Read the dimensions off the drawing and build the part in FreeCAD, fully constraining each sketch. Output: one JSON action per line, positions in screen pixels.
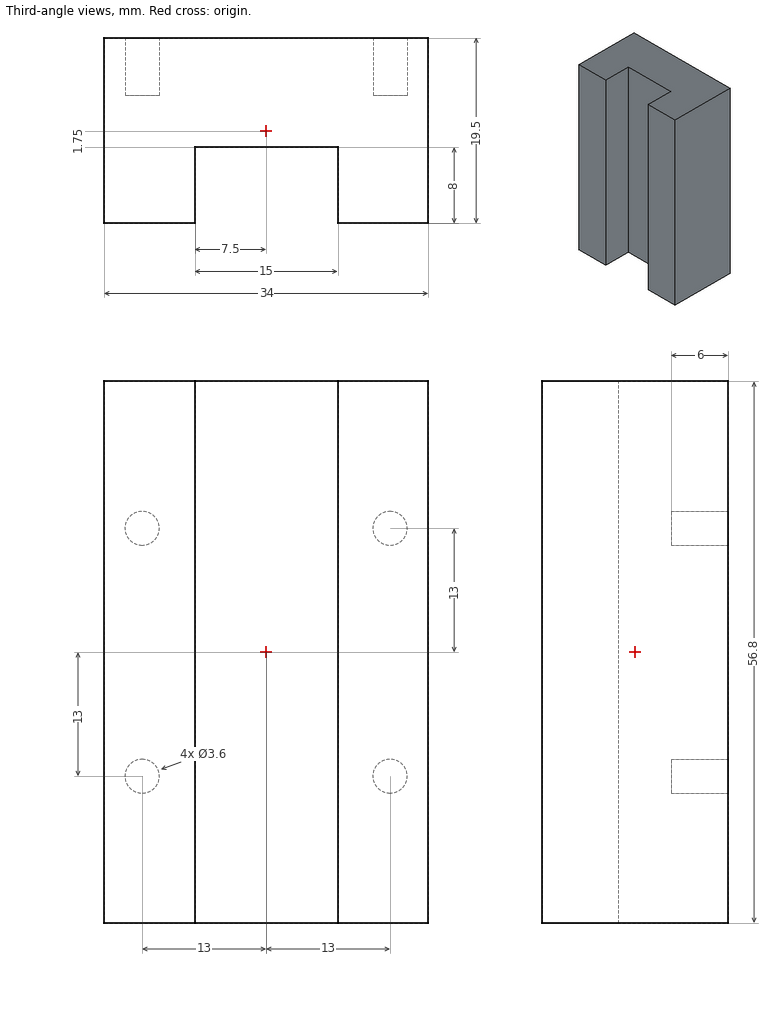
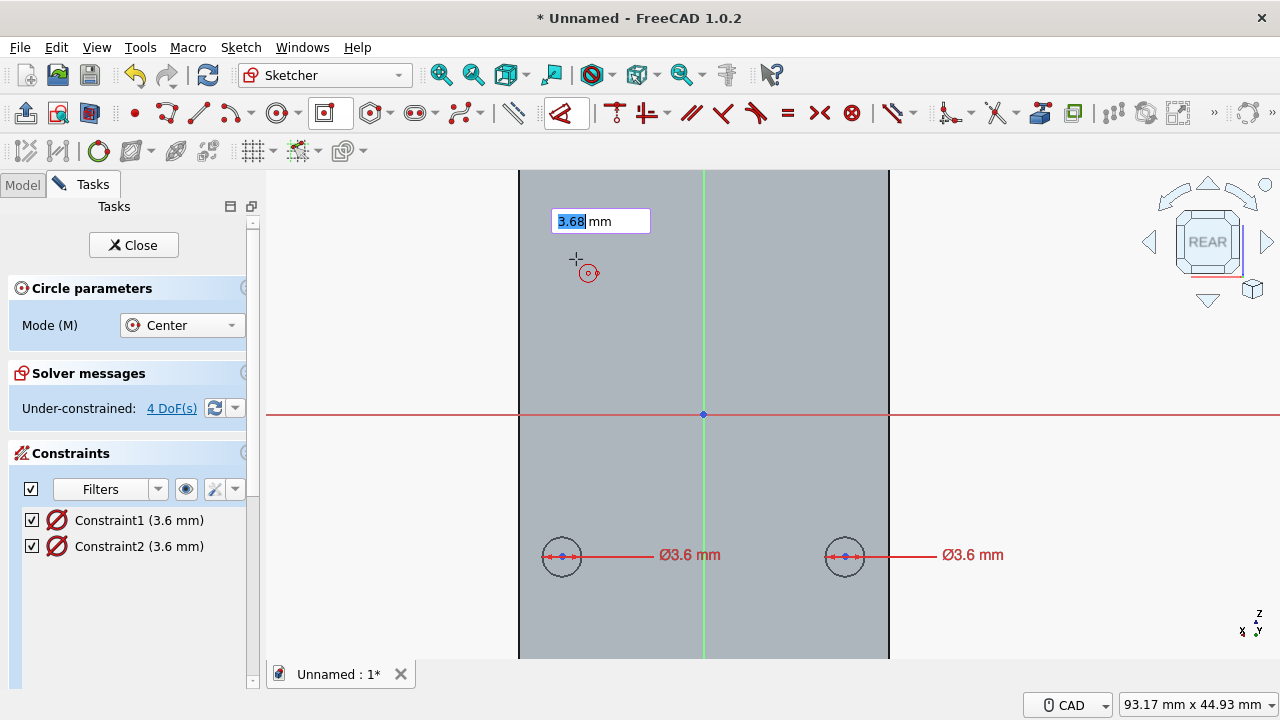
{"action": "type", "text": "3.6"}
{"action": "key", "text": "Return"}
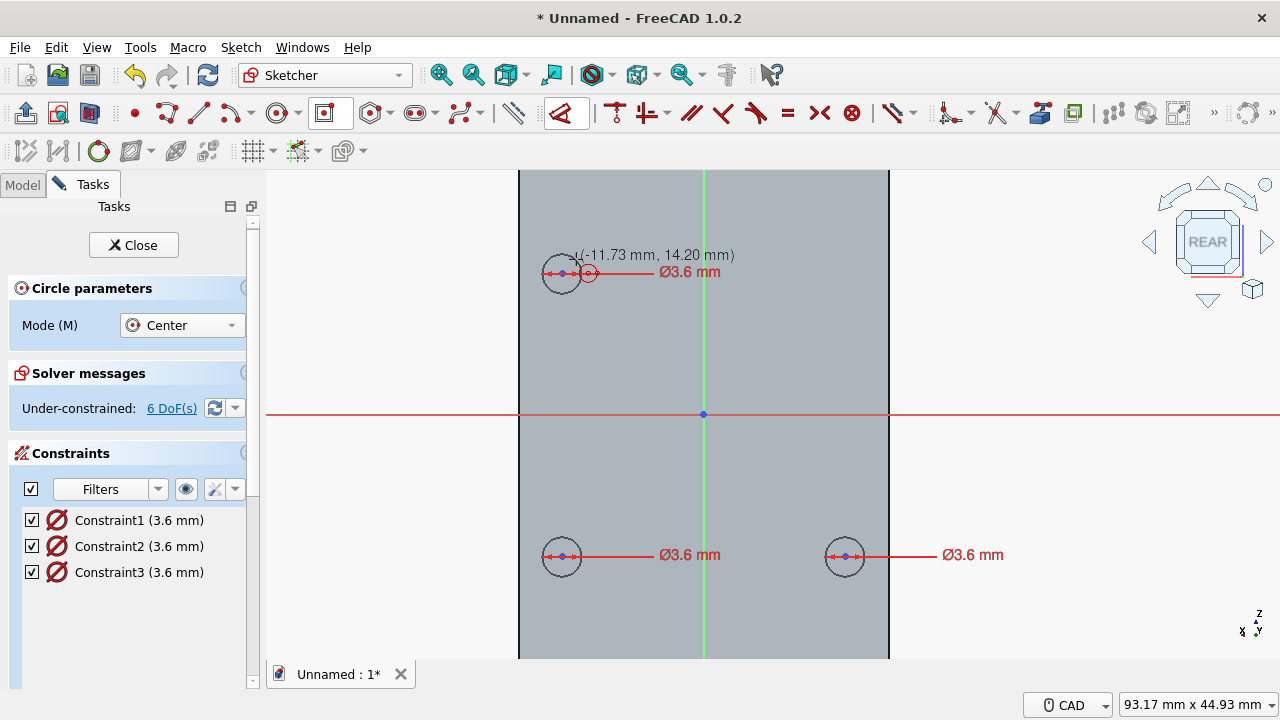
{"action": "left_click", "coordinate": [845, 273]}
{"action": "mouse_move", "coordinate": [859, 259]}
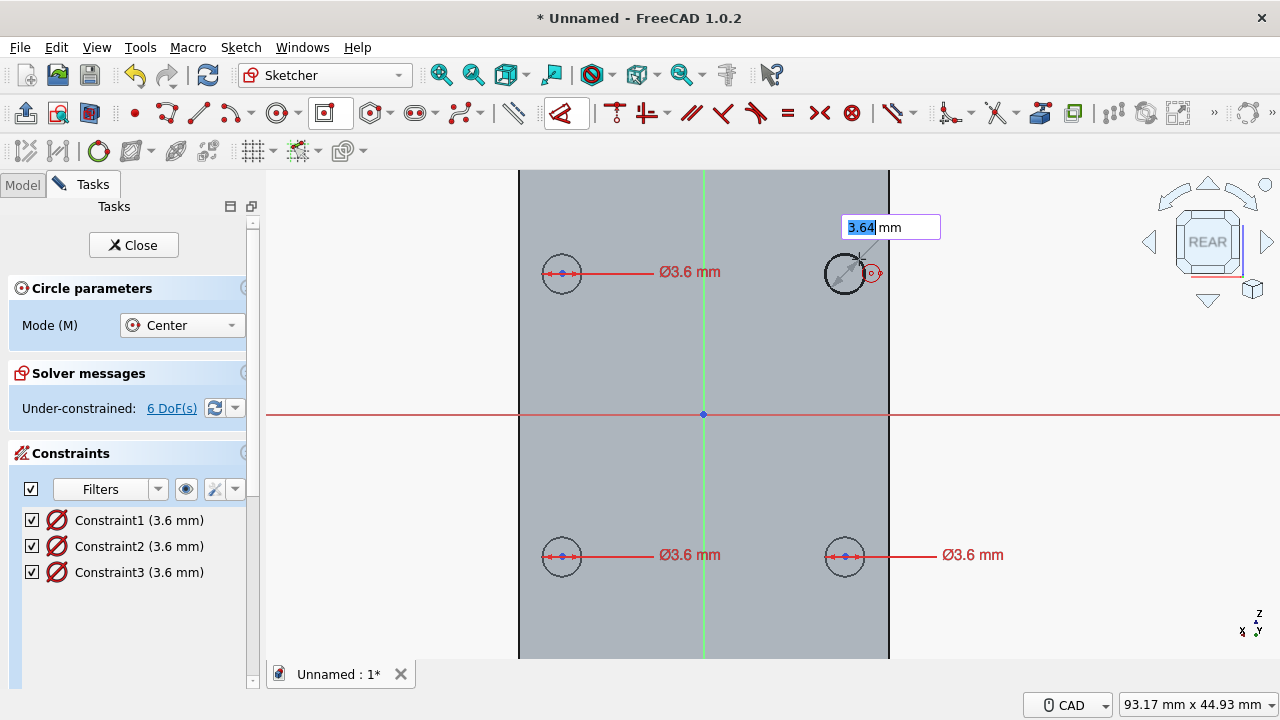
{"action": "type", "text": "3.6"}
{"action": "key", "text": "Return"}
{"action": "key", "text": "Escape"}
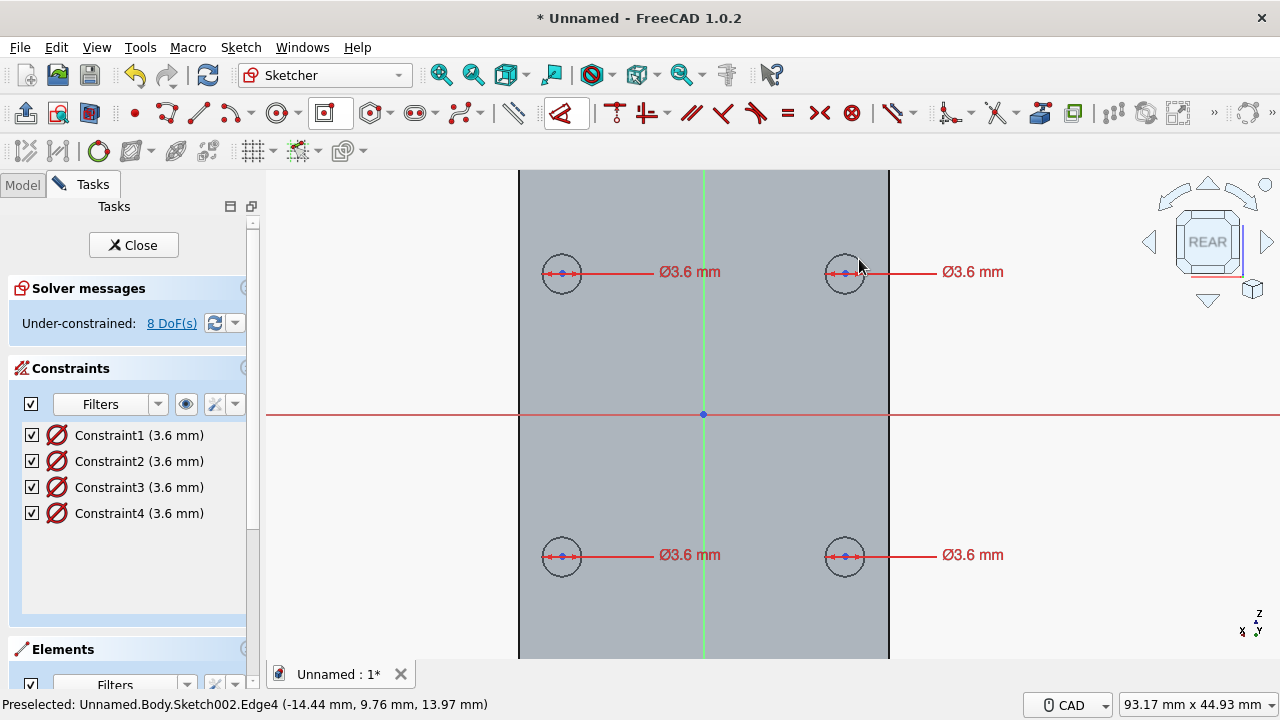
{"action": "left_click", "coordinate": [845, 557]}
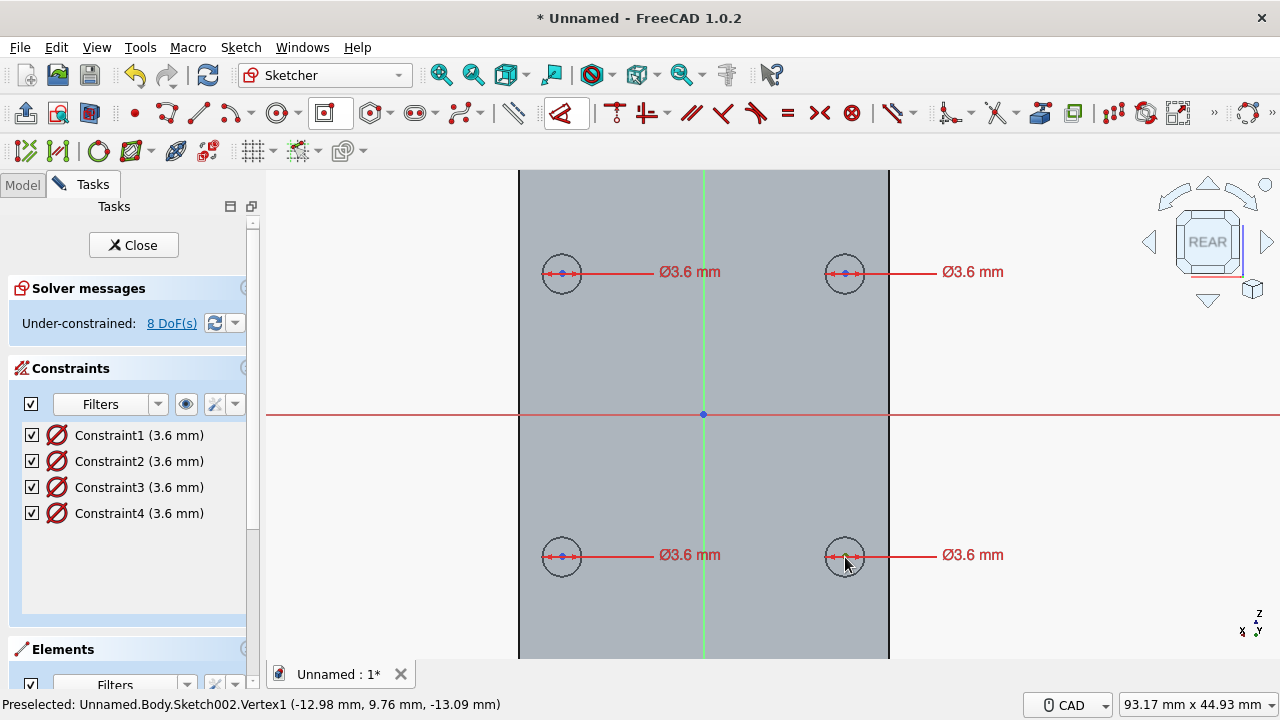
{"action": "left_click", "coordinate": [562, 557]}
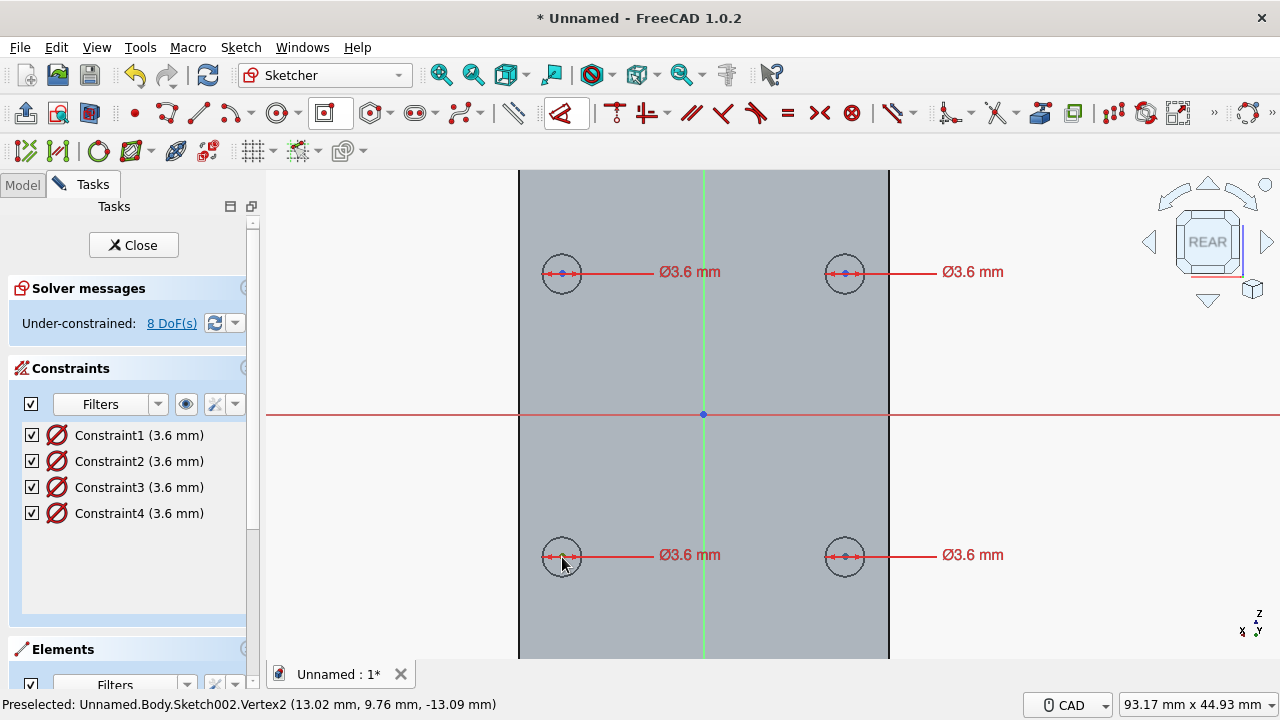
{"action": "left_click", "coordinate": [670, 114]}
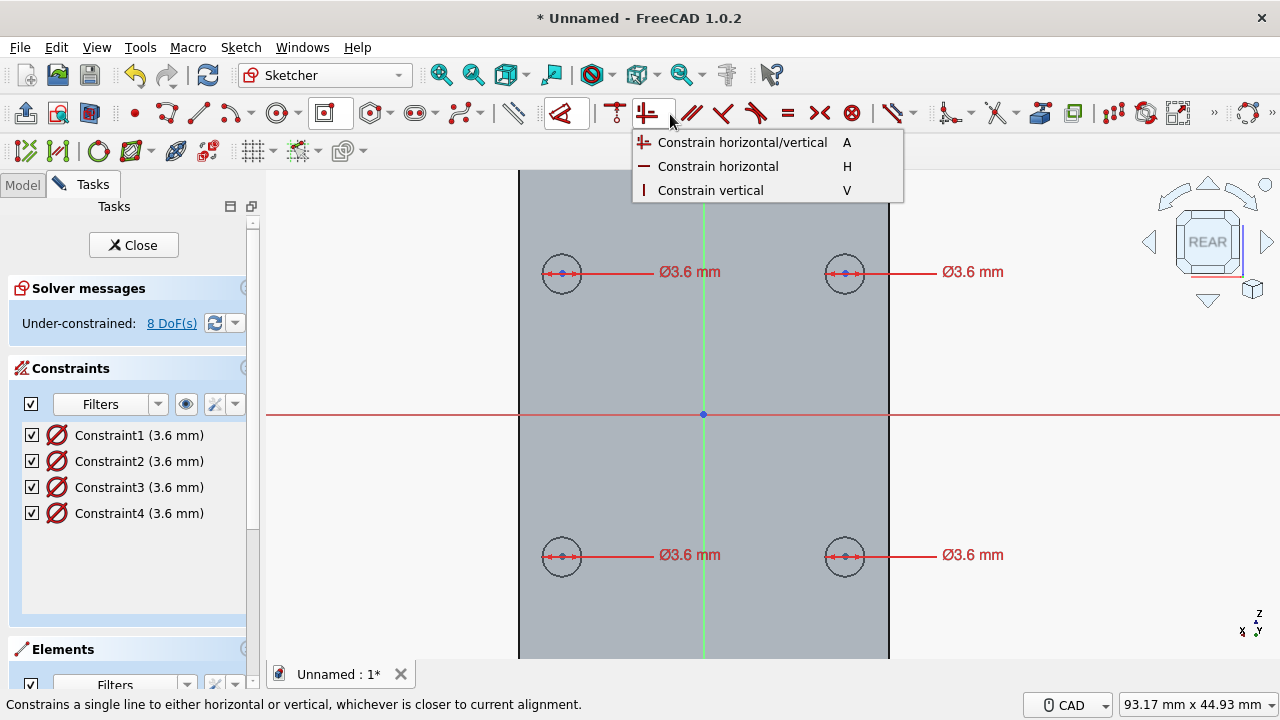
{"action": "left_click", "coordinate": [768, 166]}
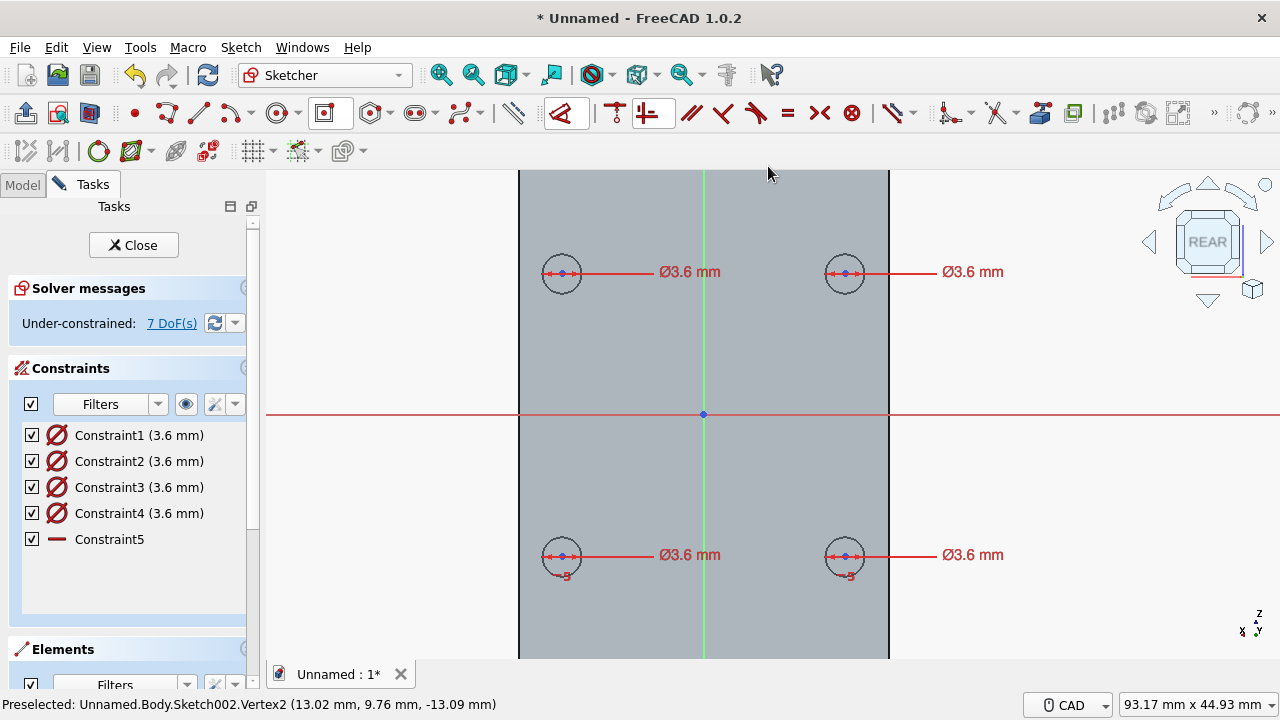
{"action": "left_click", "coordinate": [562, 557]}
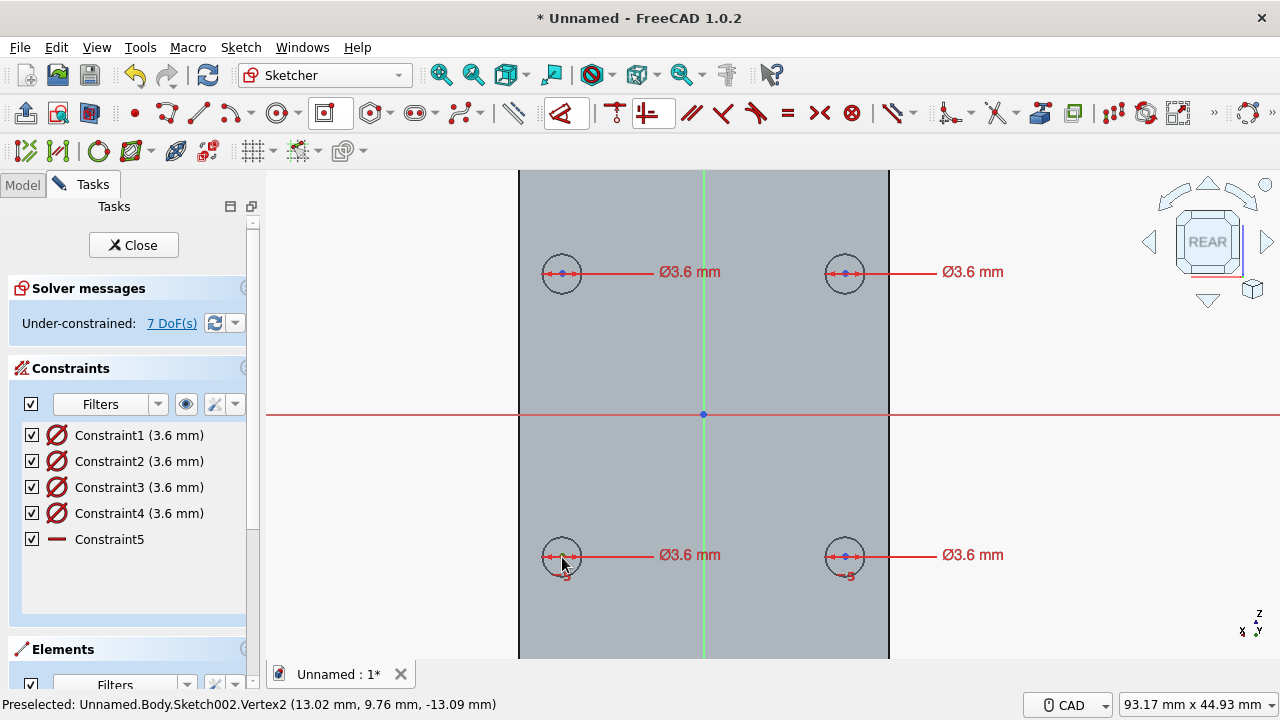
{"action": "left_click", "coordinate": [562, 274]}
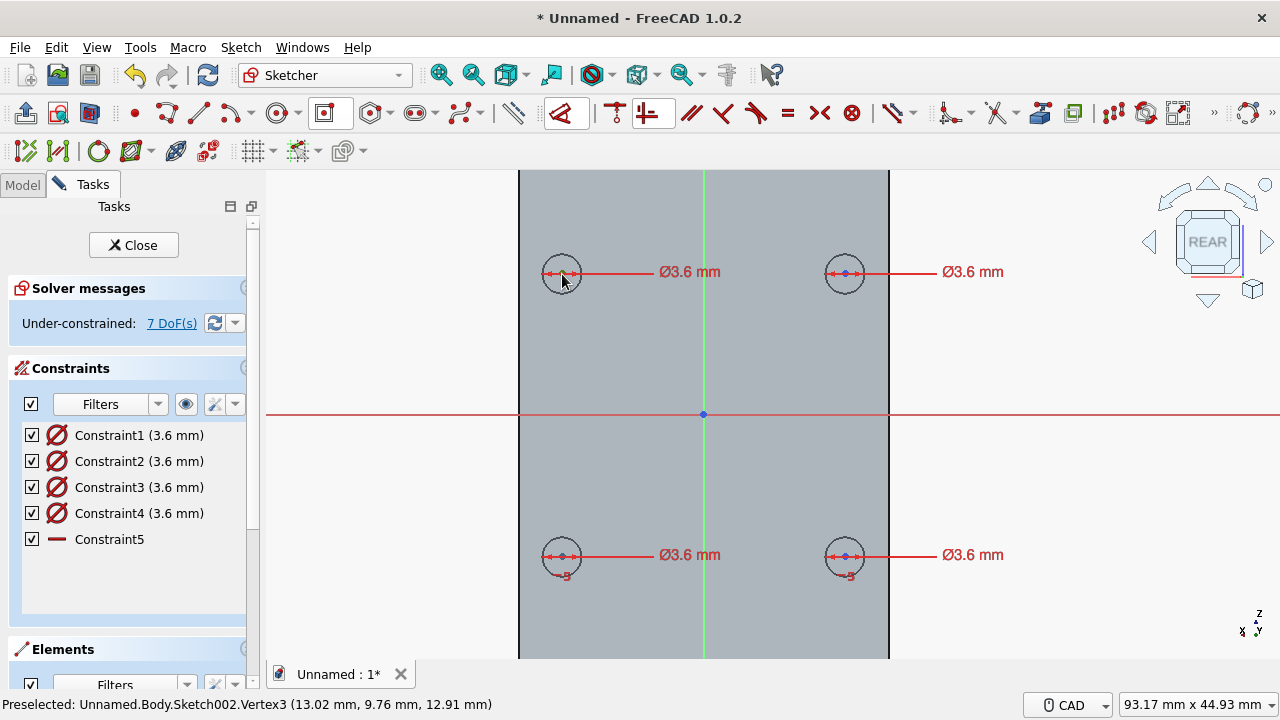
{"action": "key", "text": "v"}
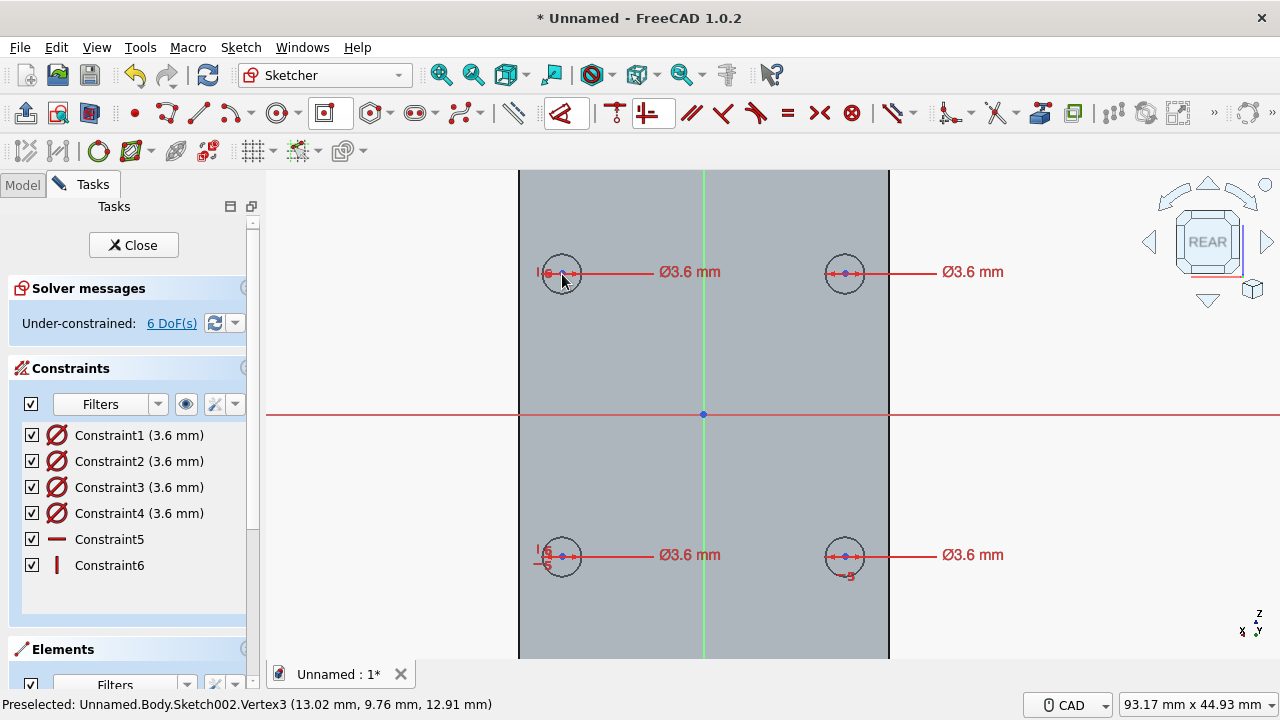
{"action": "left_click", "coordinate": [845, 557]}